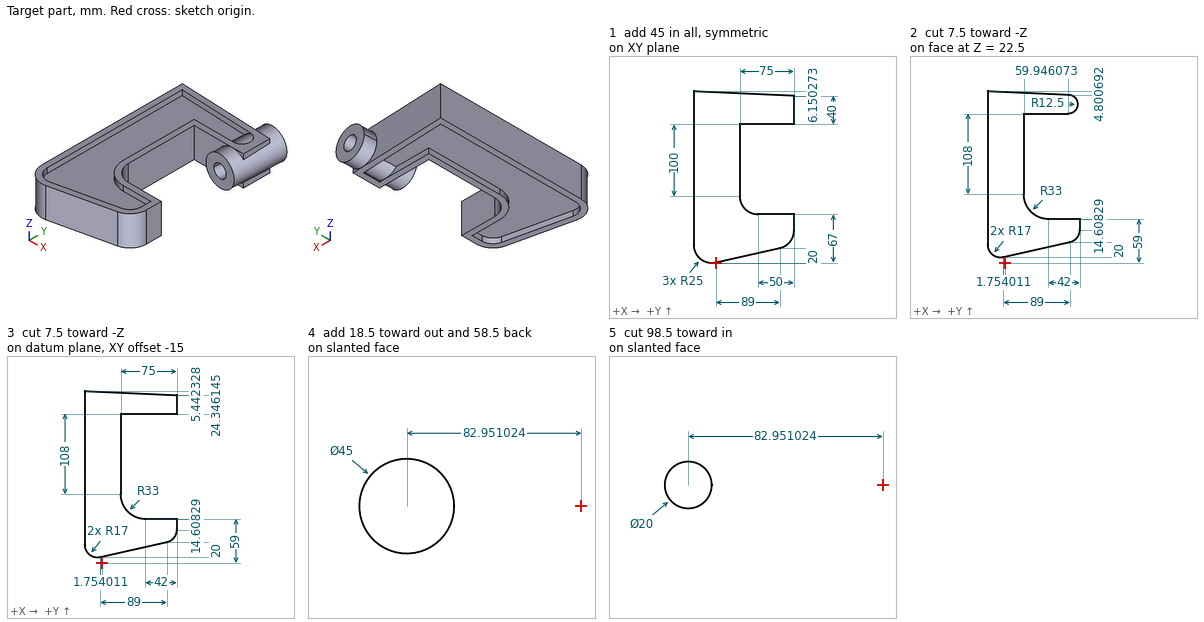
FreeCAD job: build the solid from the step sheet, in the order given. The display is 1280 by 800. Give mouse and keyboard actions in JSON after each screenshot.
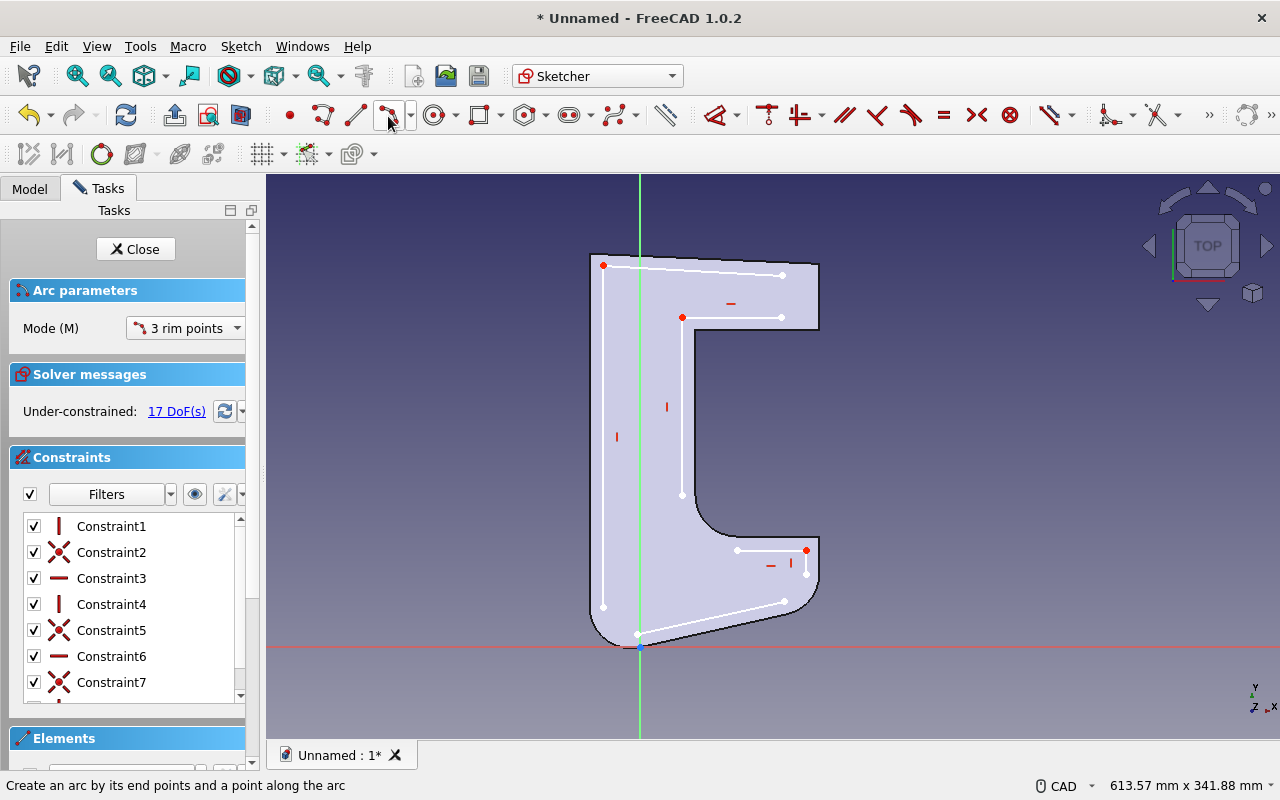
{"action": "left_click", "coordinate": [784, 602]}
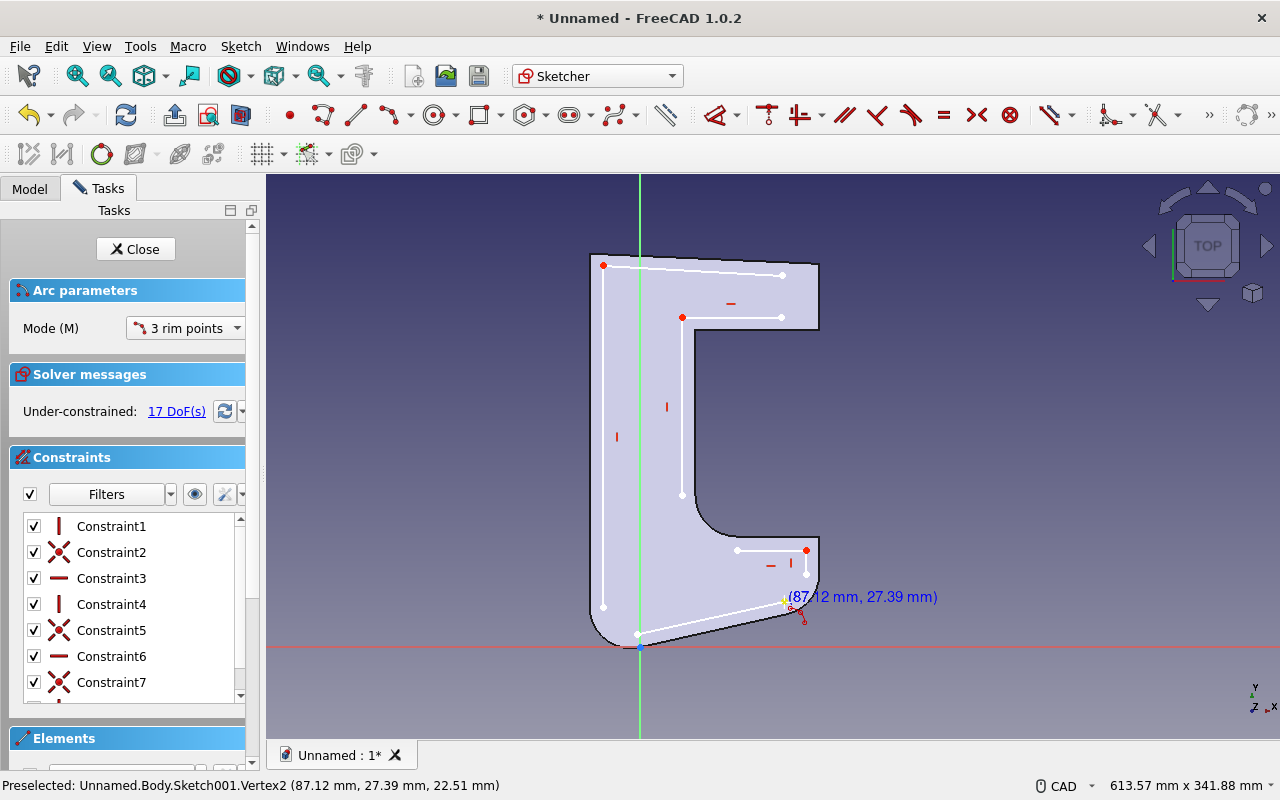
{"action": "scroll", "coordinate": [806, 574], "scroll_direction": "up", "scroll_amount": 2}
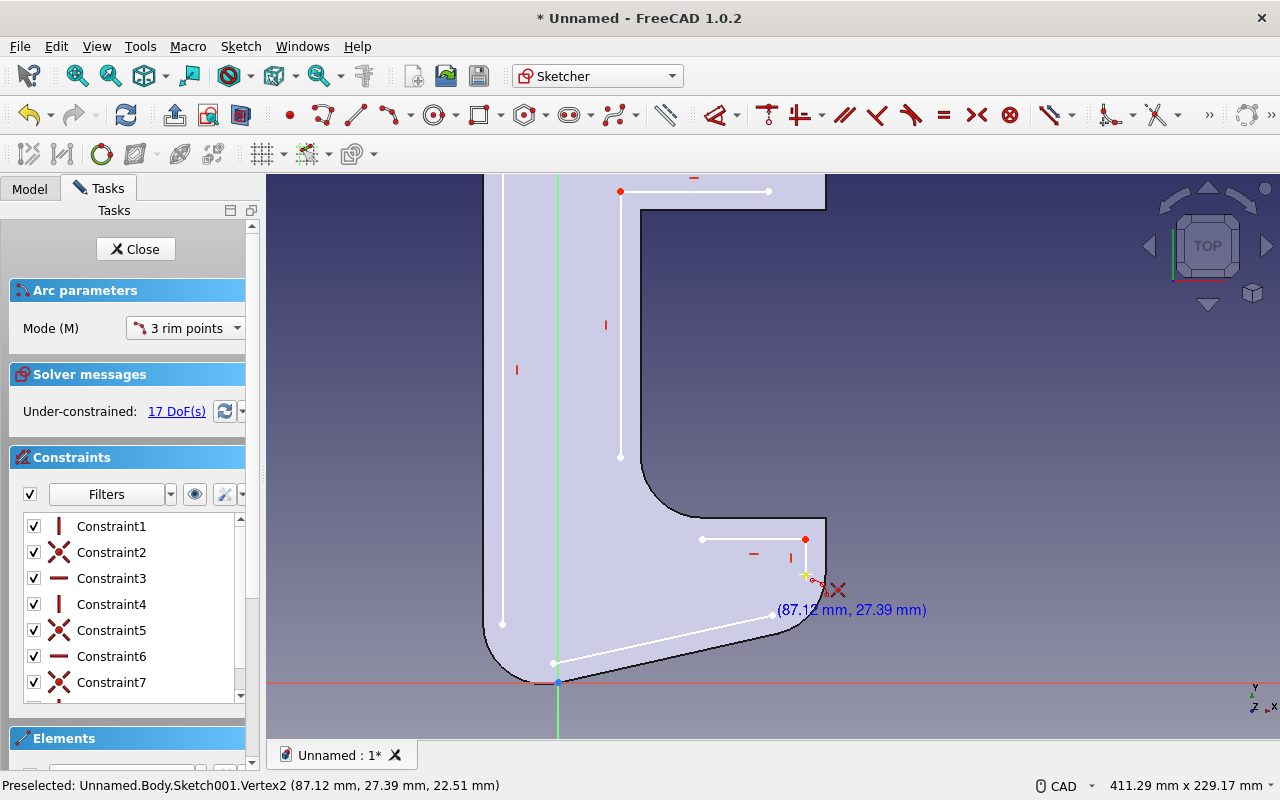
{"action": "left_click", "coordinate": [806, 575]}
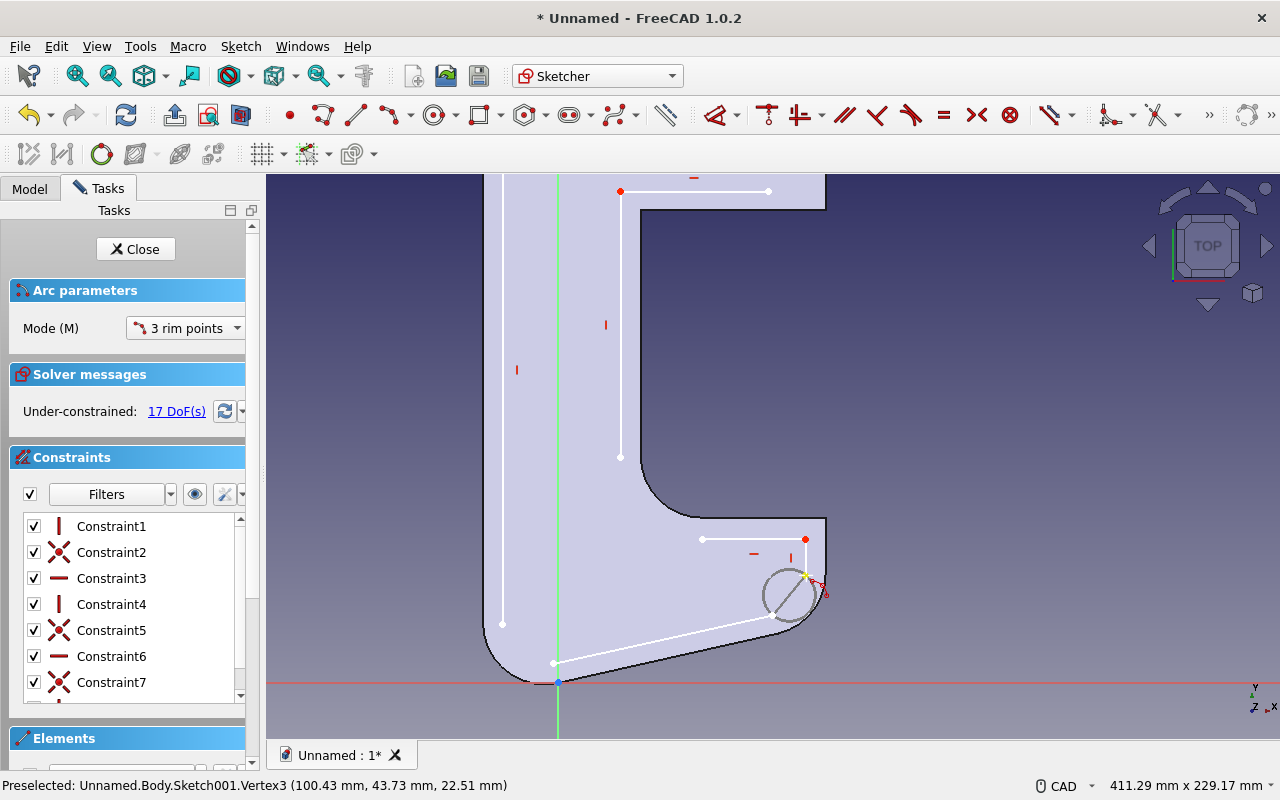
{"action": "scroll", "coordinate": [797, 600], "scroll_direction": "up", "scroll_amount": 3}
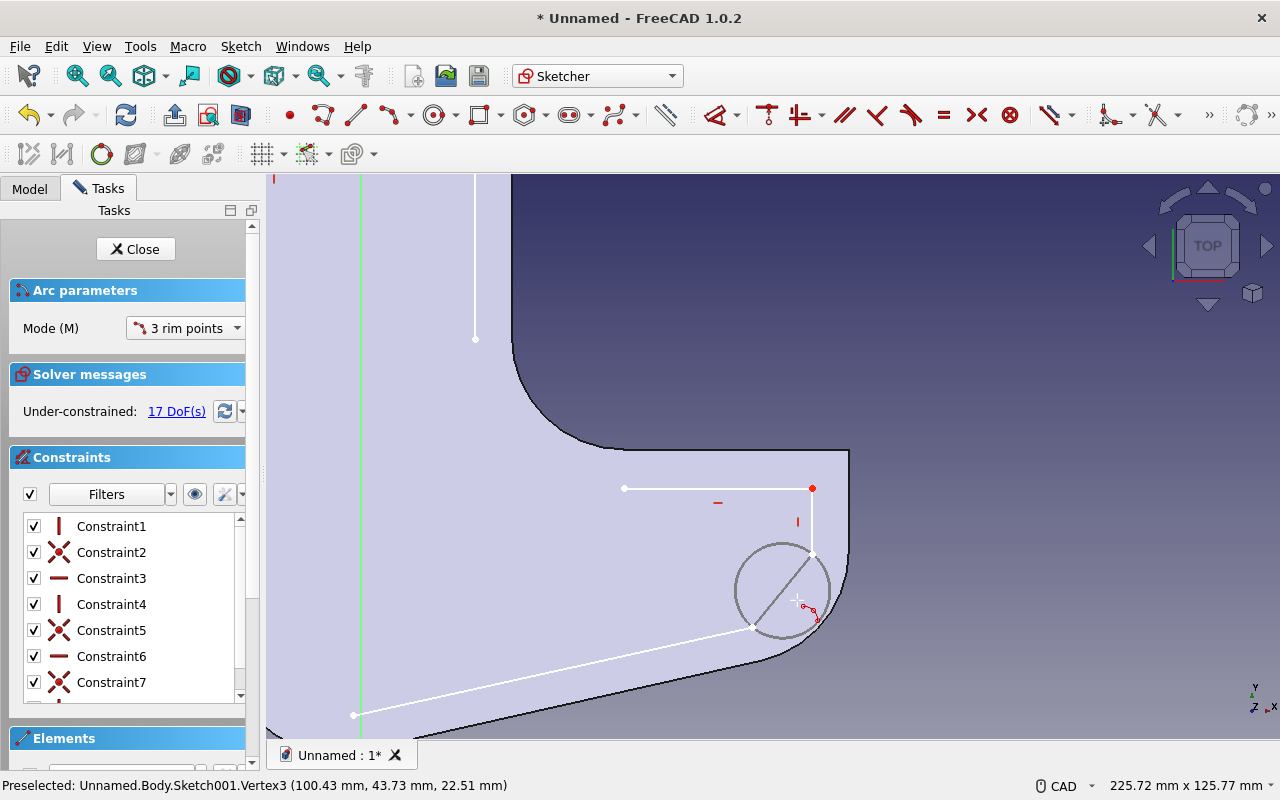
{"action": "left_click", "coordinate": [796, 599]}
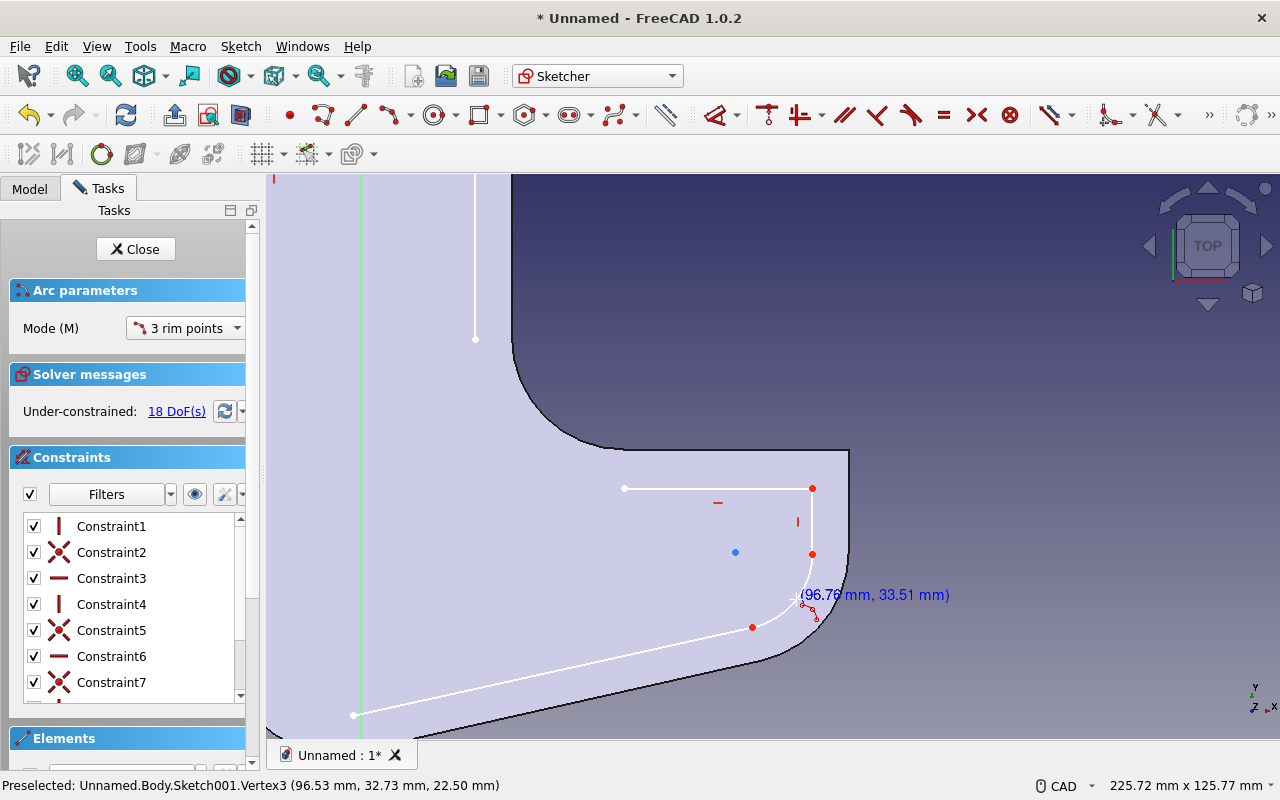
{"action": "left_click", "coordinate": [625, 489]}
{"action": "left_click", "coordinate": [475, 339]}
{"action": "left_click", "coordinate": [519, 442]}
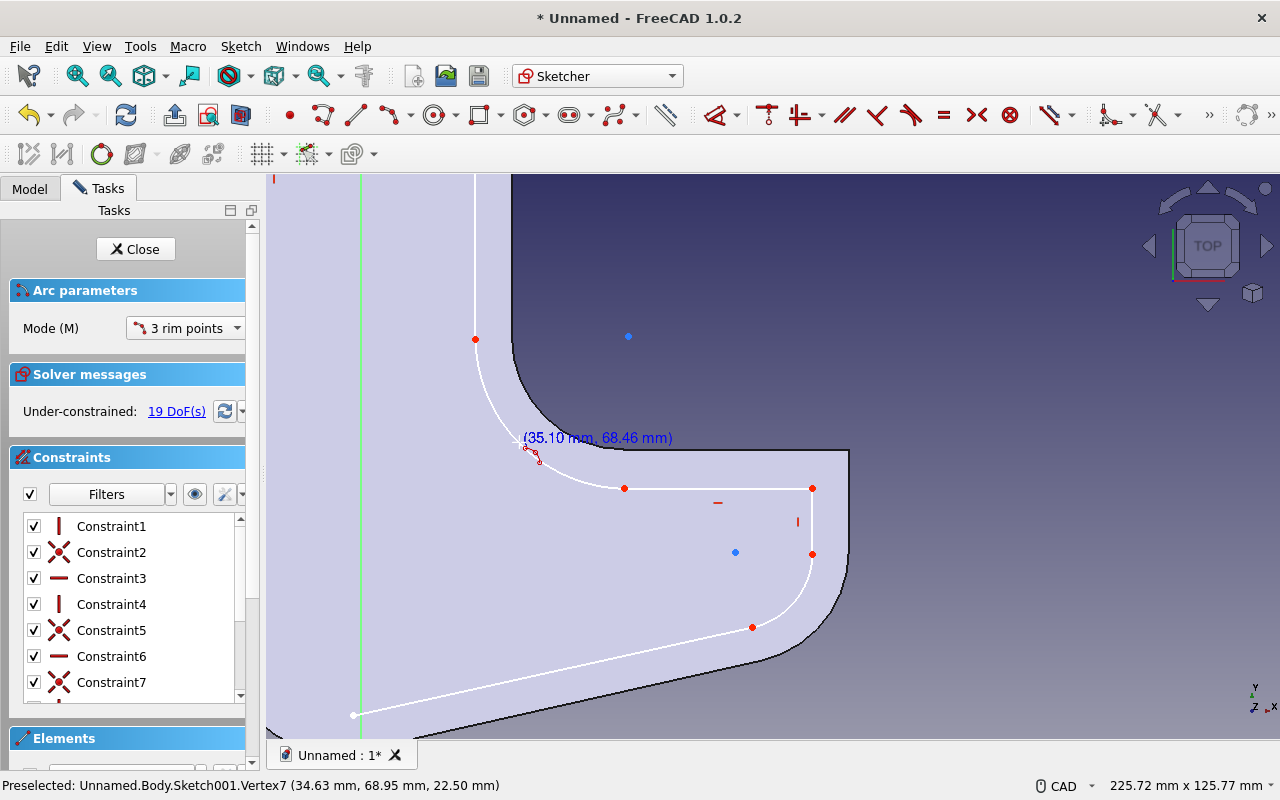
{"action": "scroll", "coordinate": [802, 586], "scroll_direction": "down", "scroll_amount": 5}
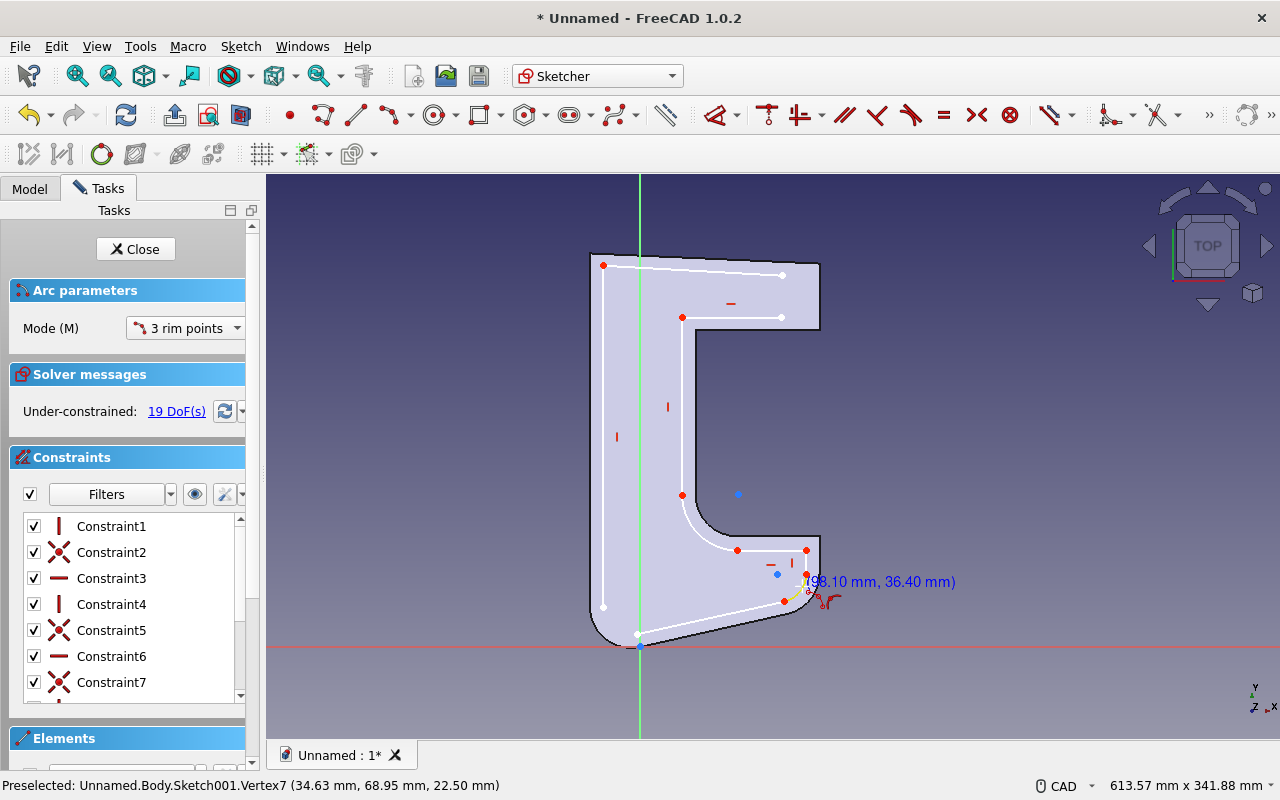
{"action": "left_click", "coordinate": [781, 318]}
{"action": "left_click", "coordinate": [782, 276]}
{"action": "left_click", "coordinate": [802, 296]}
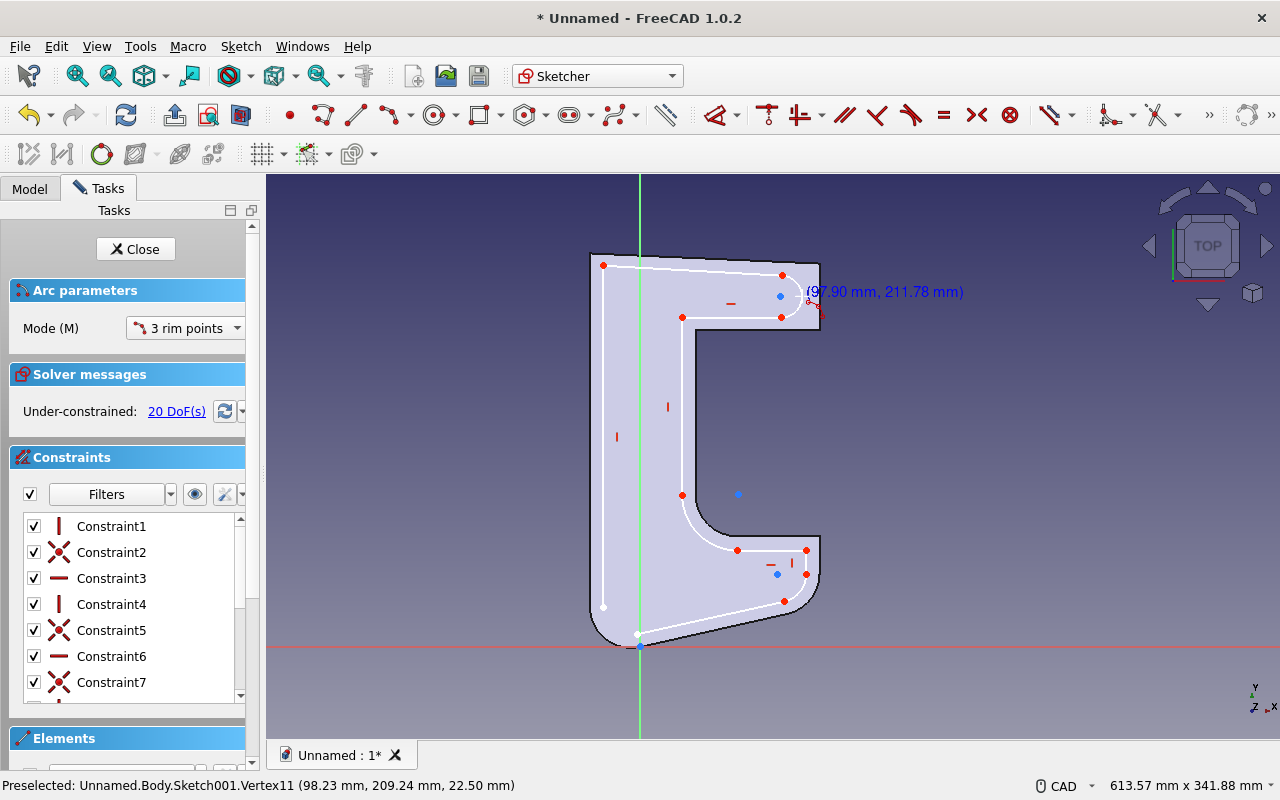
{"action": "left_click", "coordinate": [603, 608]}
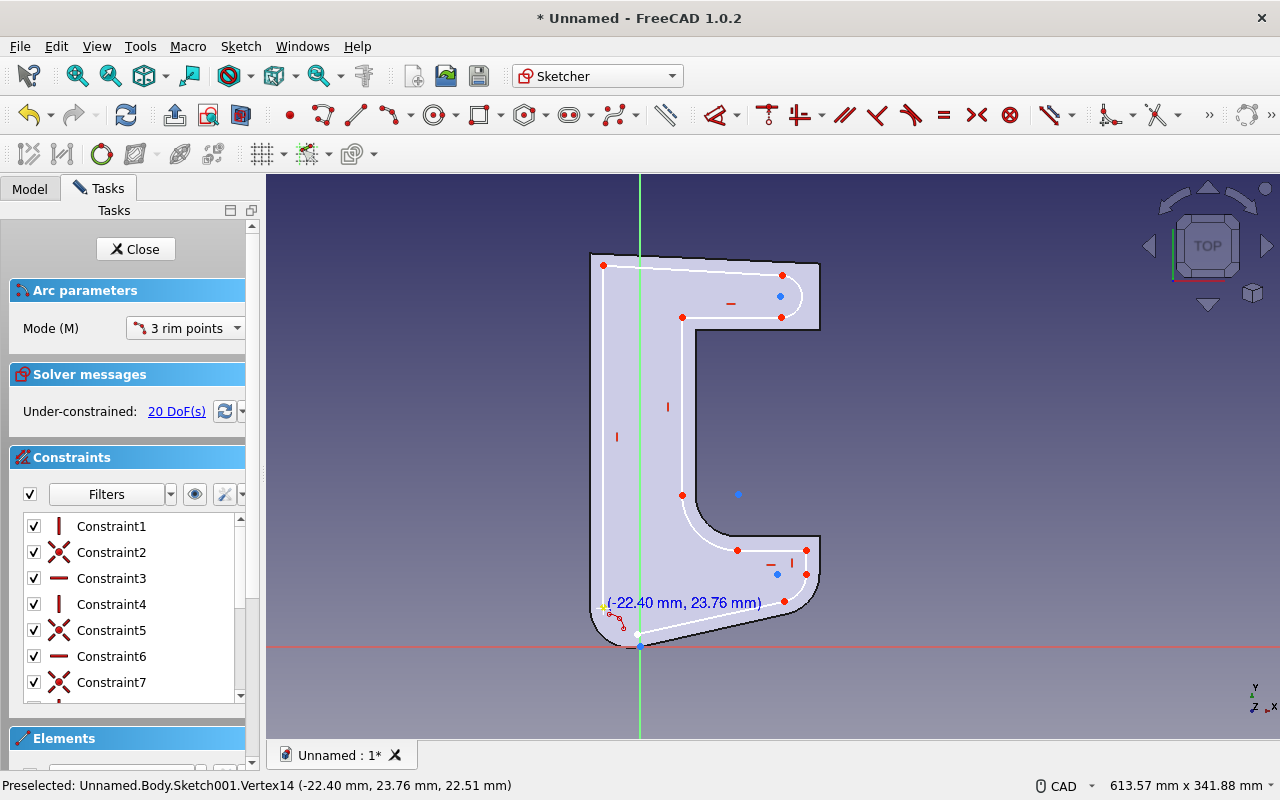
{"action": "scroll", "coordinate": [637, 634], "scroll_direction": "up", "scroll_amount": 9}